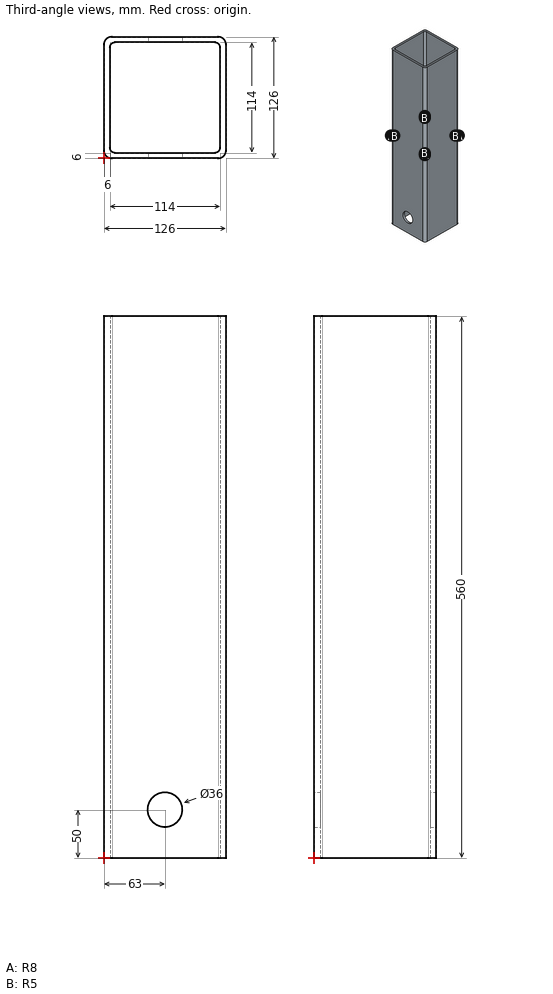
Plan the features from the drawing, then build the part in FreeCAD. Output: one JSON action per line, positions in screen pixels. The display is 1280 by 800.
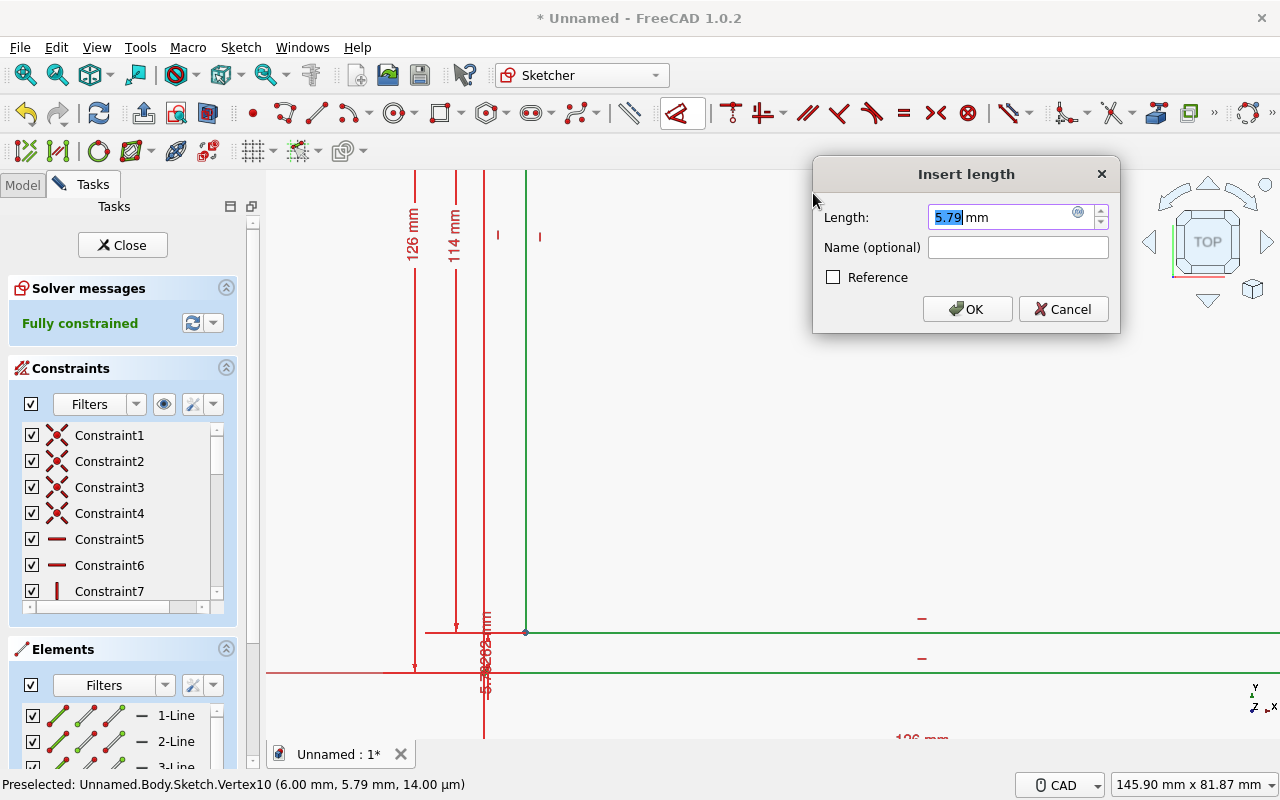
{"action": "type", "text": "6"}
{"action": "key", "text": "Return"}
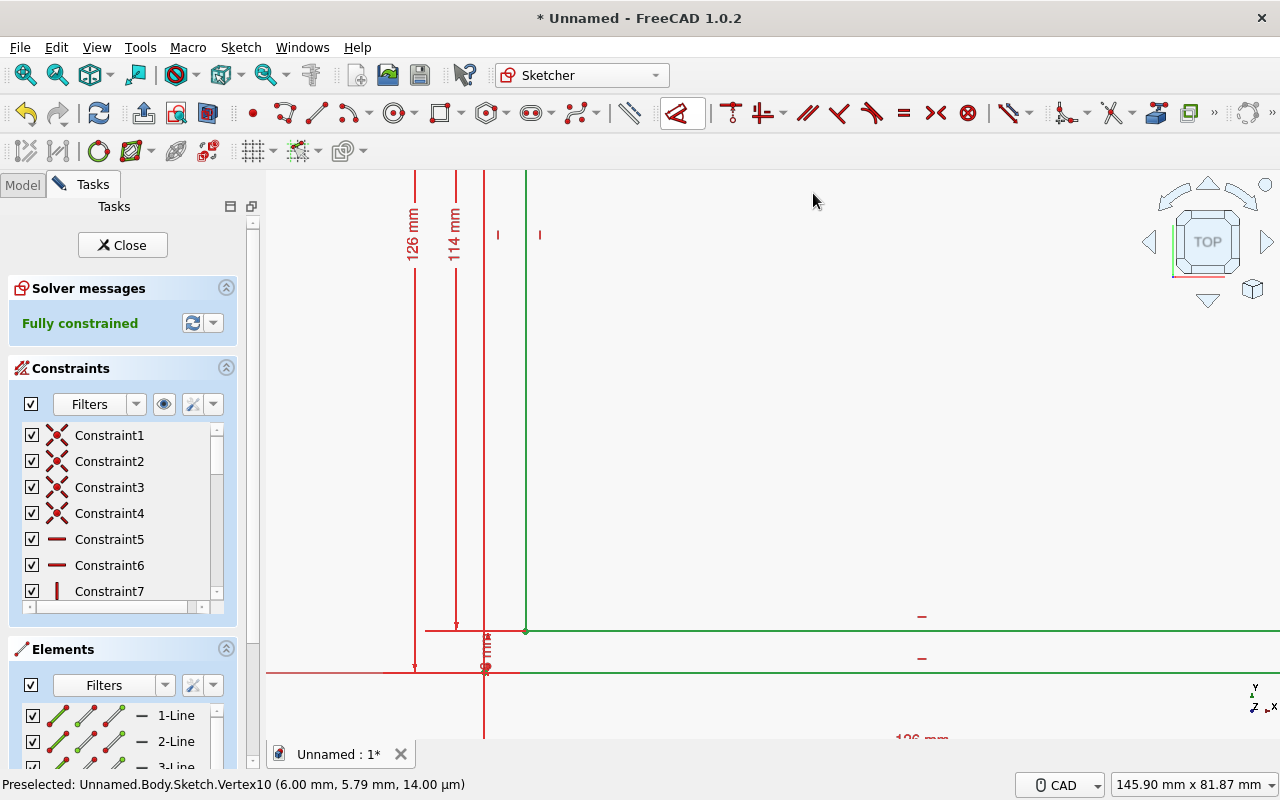
{"action": "left_click", "coordinate": [123, 245]}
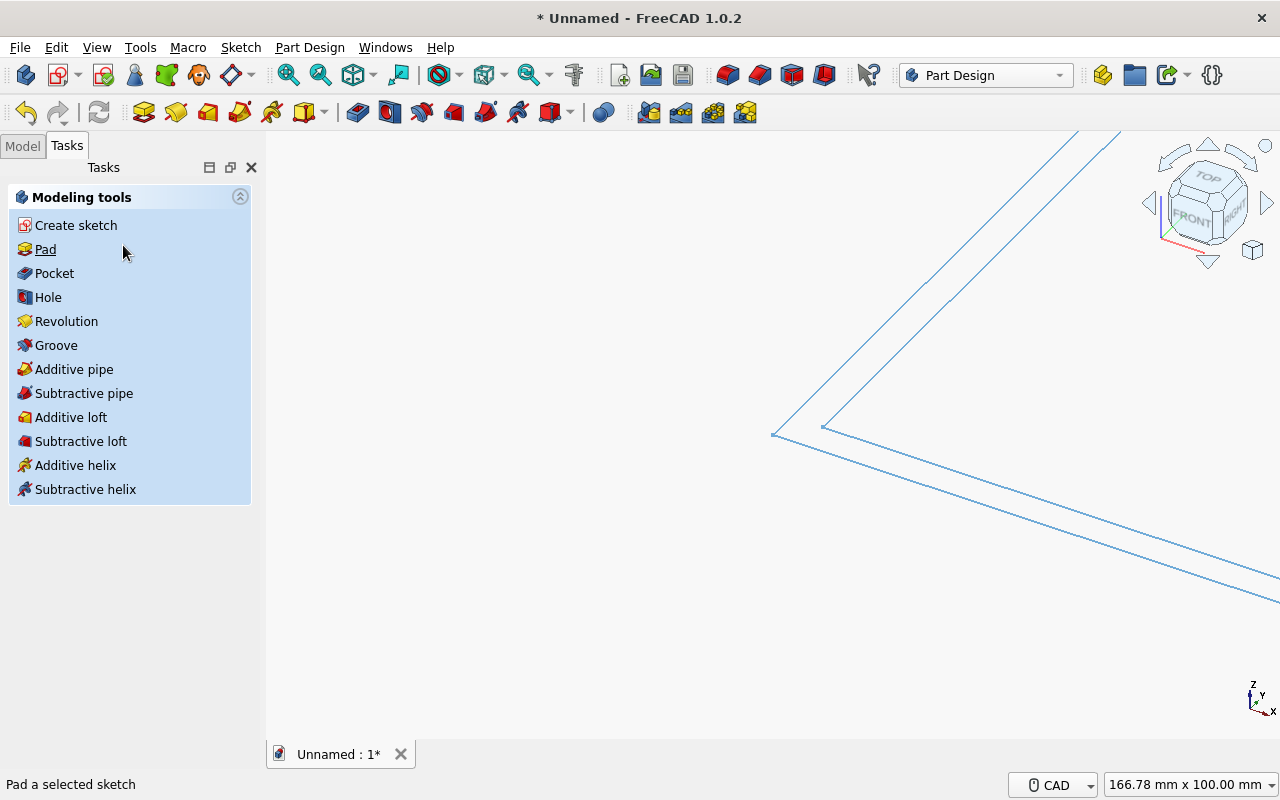
{"action": "left_click", "coordinate": [144, 112]}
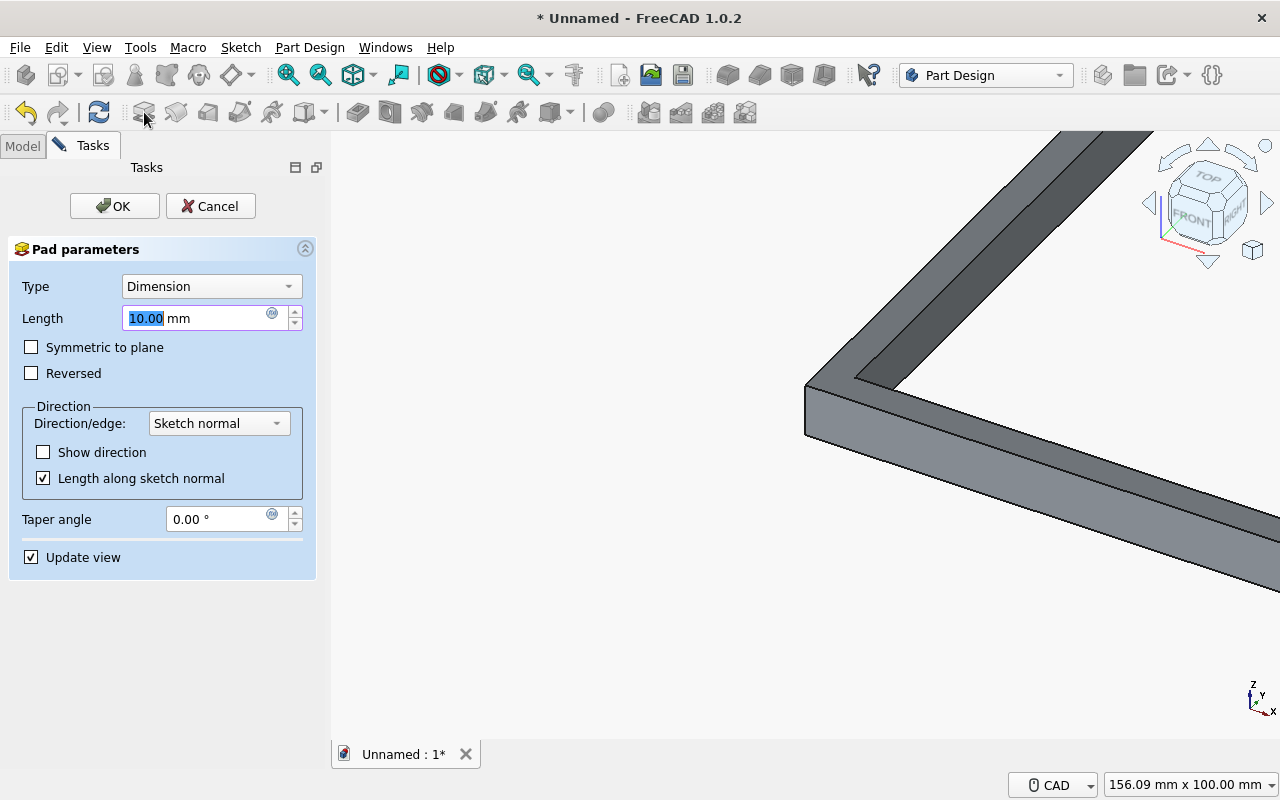
{"action": "type", "text": "560"}
{"action": "key", "text": "Tab"}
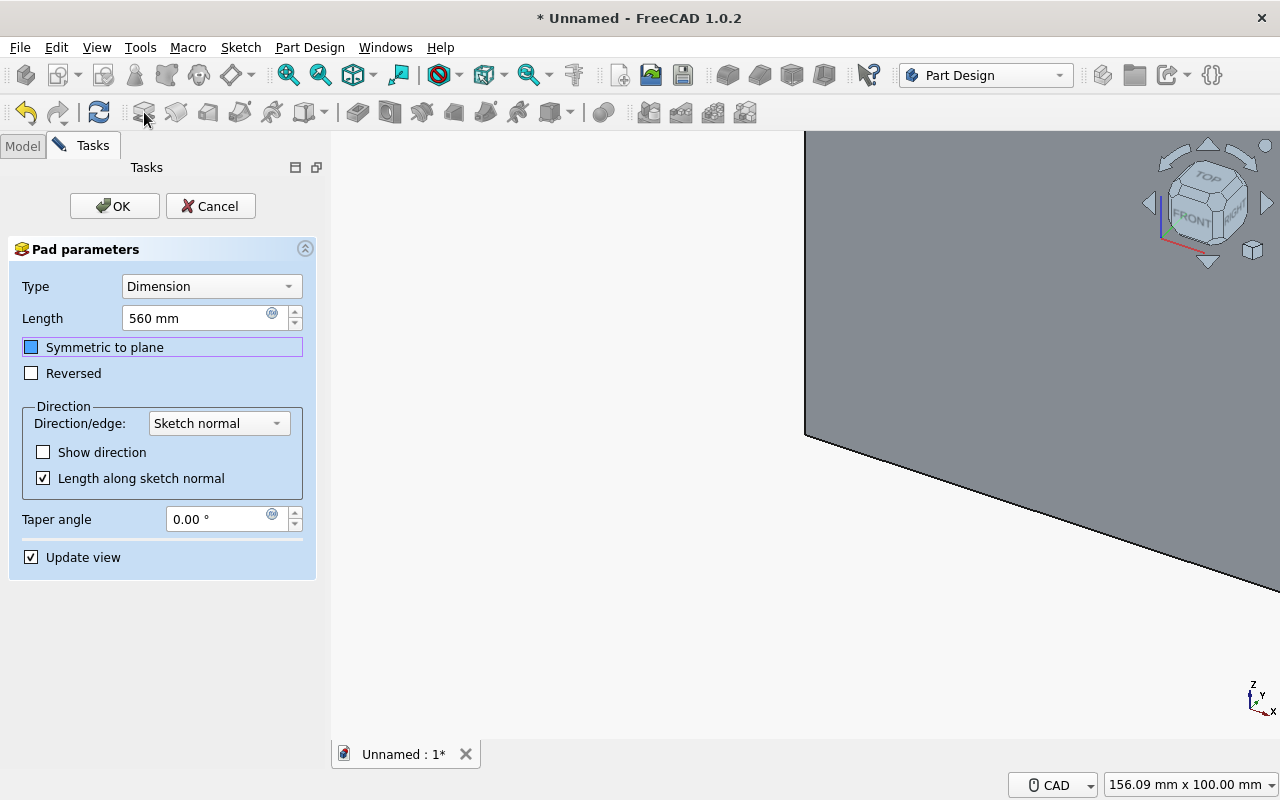
{"action": "left_click", "coordinate": [115, 206]}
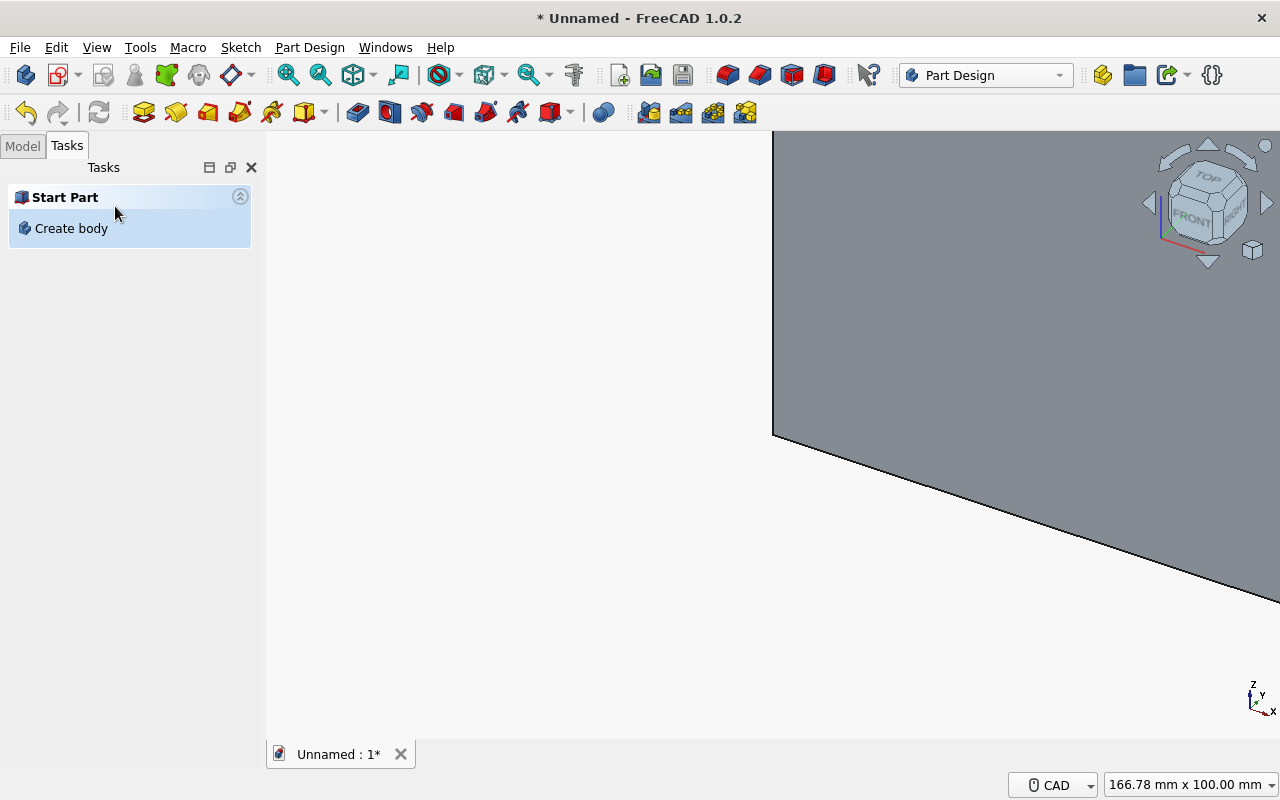
{"action": "left_click", "coordinate": [290, 76]}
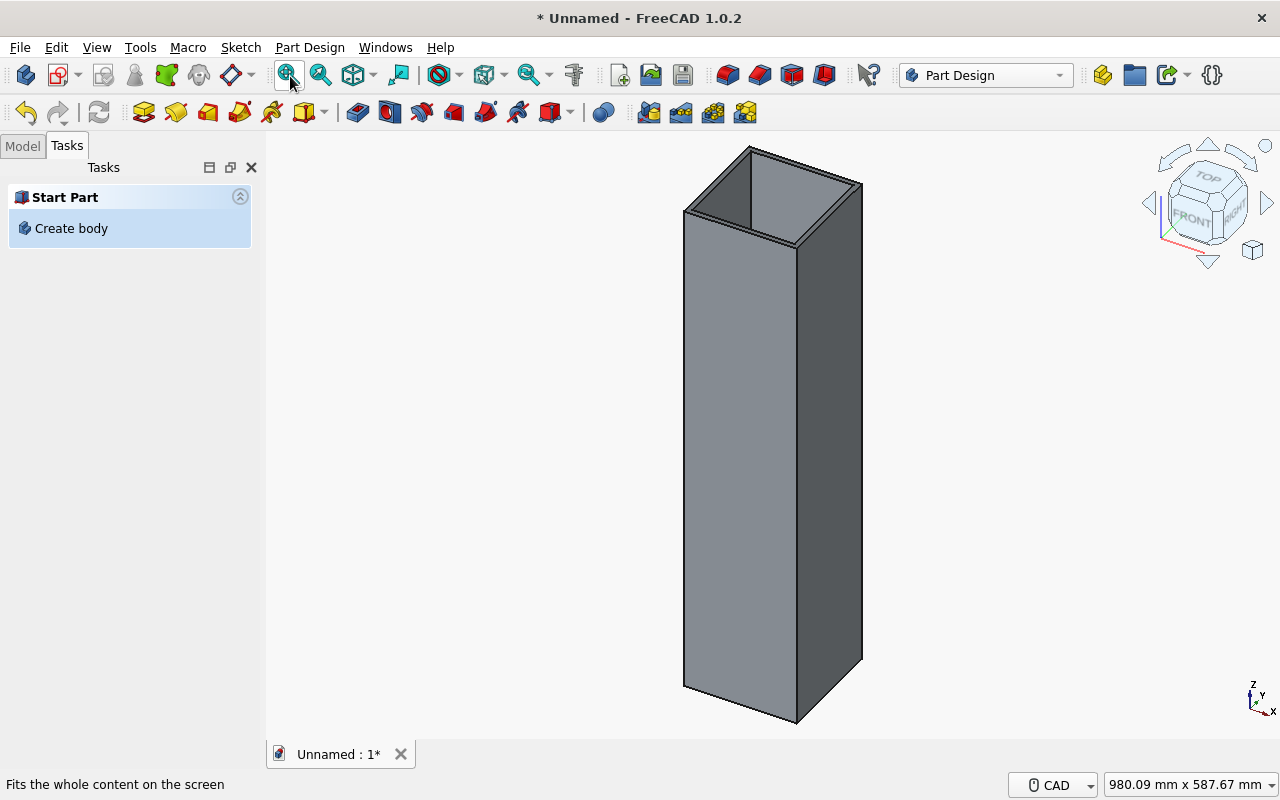
{"action": "left_click", "coordinate": [797, 485]}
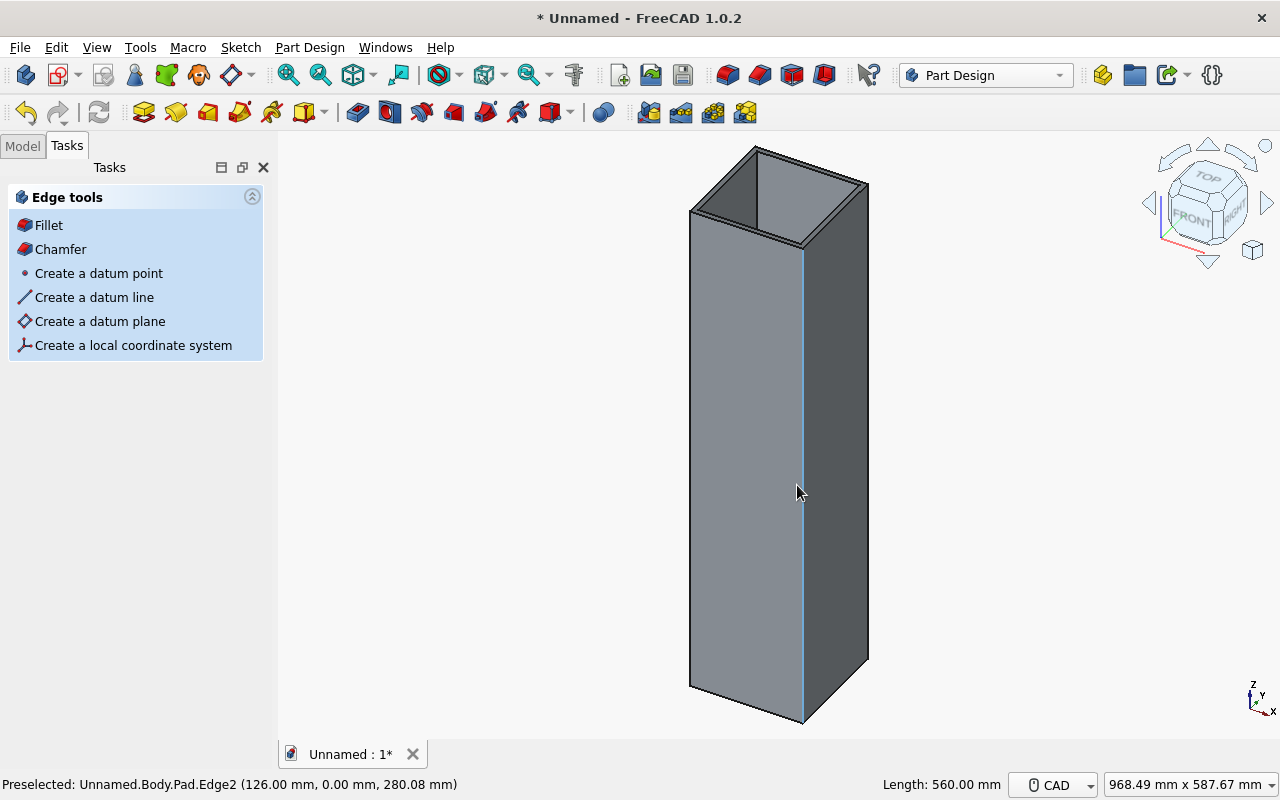
{"action": "key", "text": "0"}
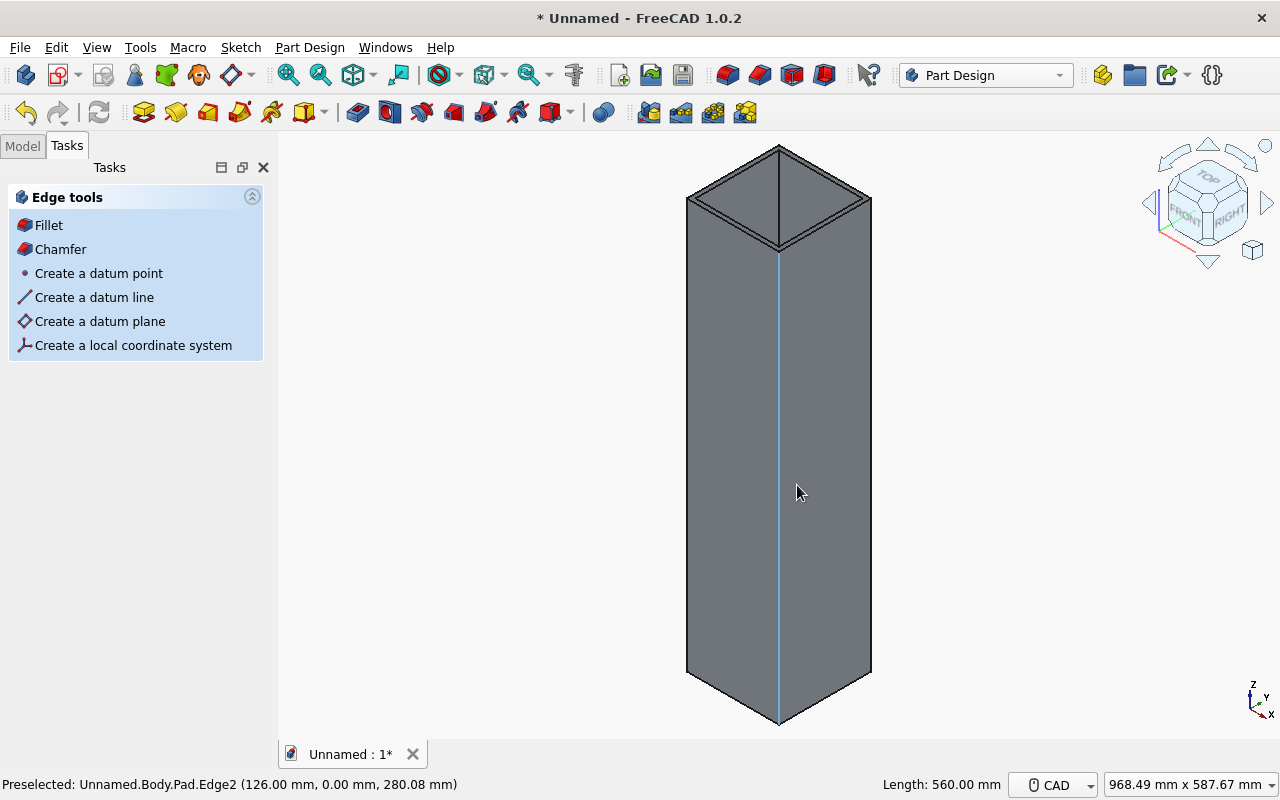
{"action": "key", "text": "2"}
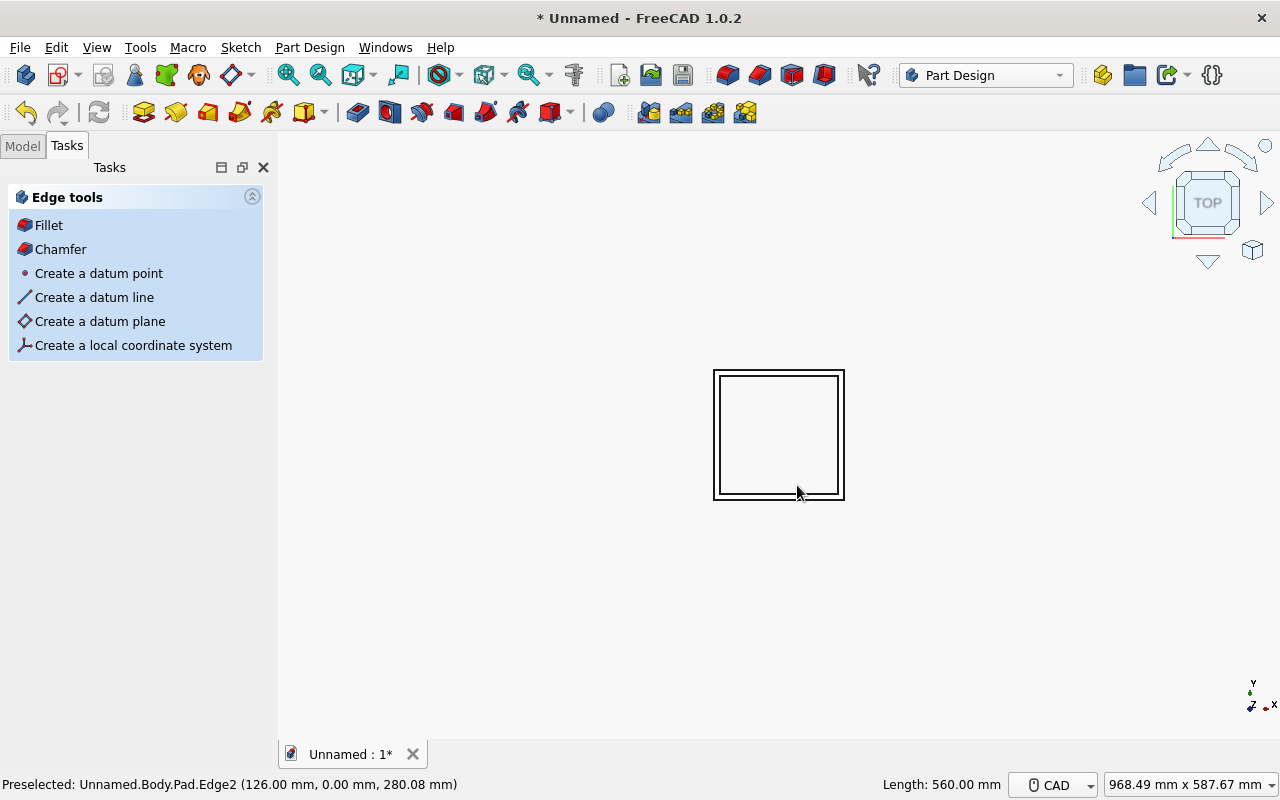
{"action": "left_click", "coordinate": [290, 76]}